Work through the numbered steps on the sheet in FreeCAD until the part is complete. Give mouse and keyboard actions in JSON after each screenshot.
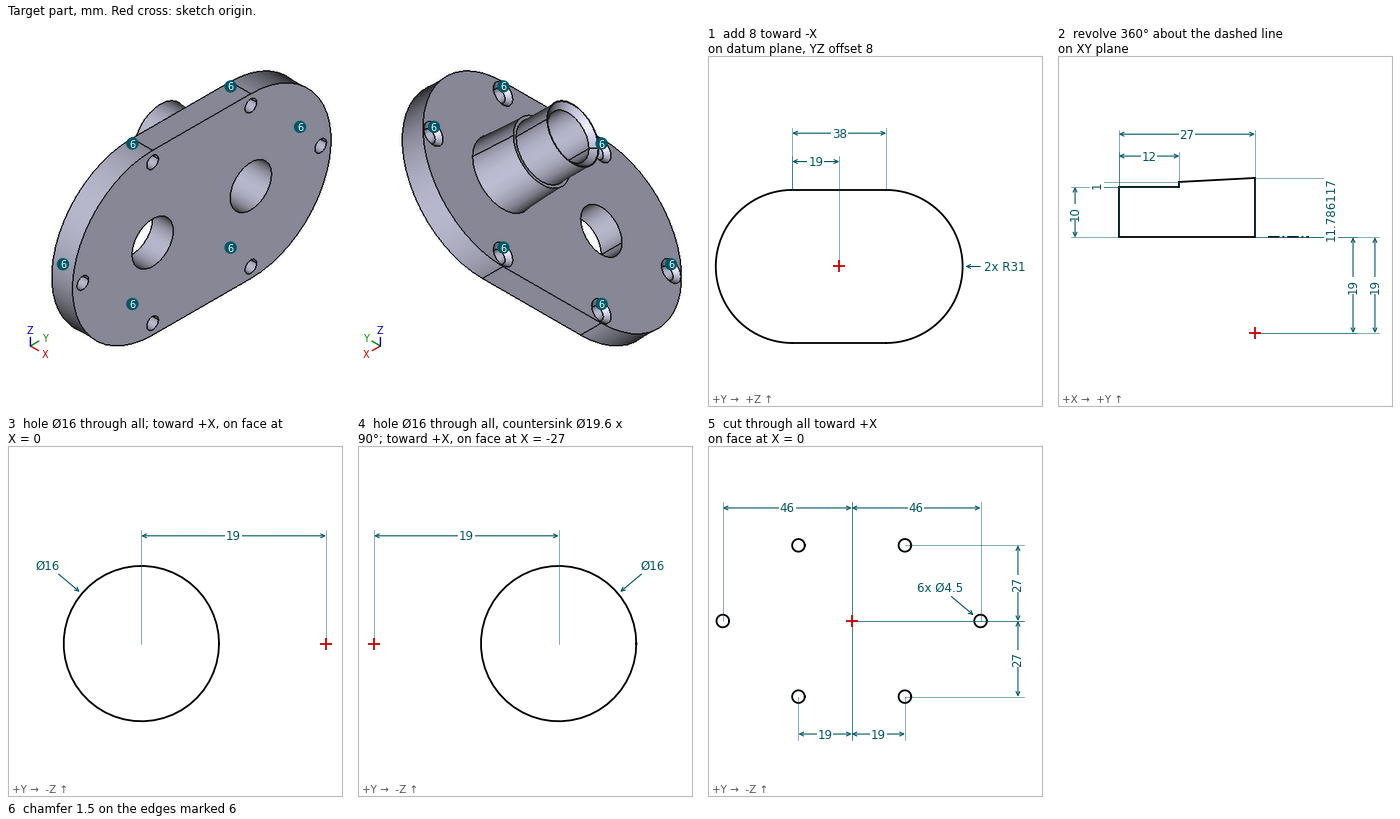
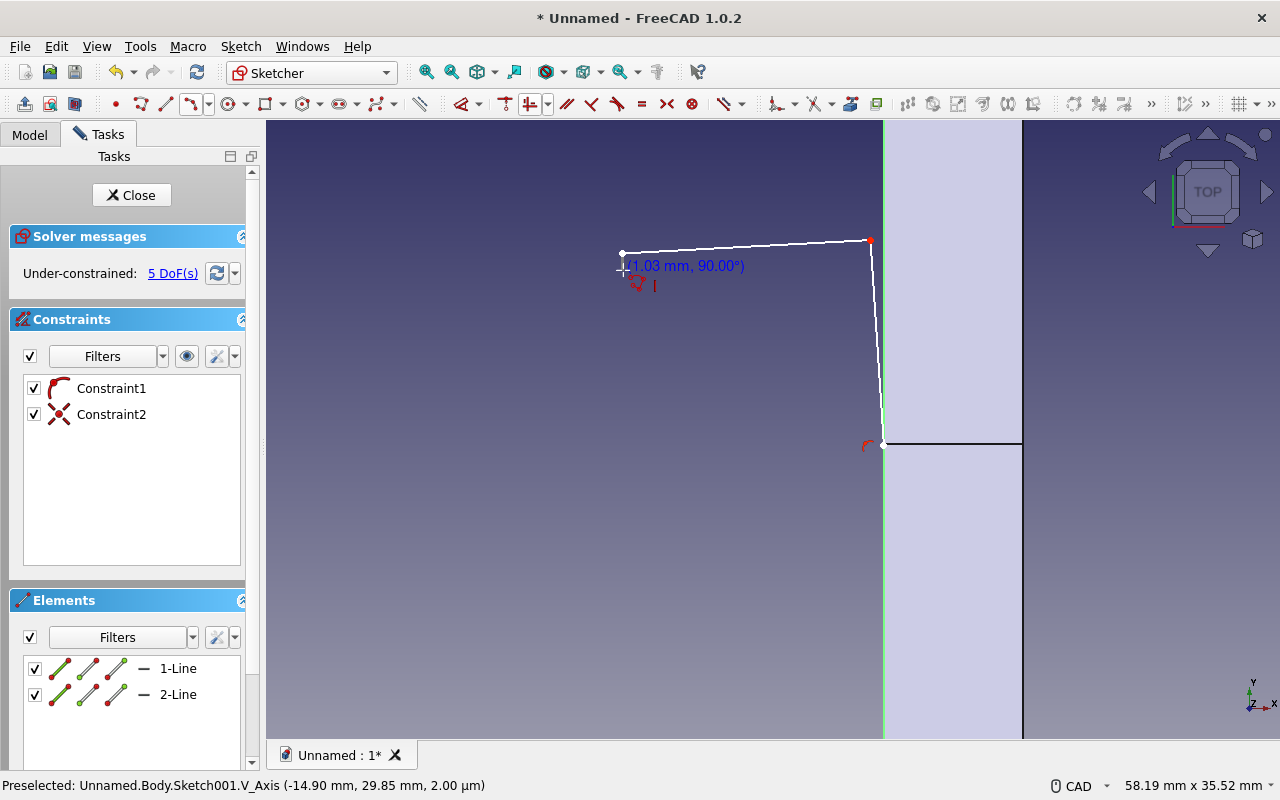
{"action": "left_click", "coordinate": [623, 270]}
{"action": "left_click", "coordinate": [413, 270]}
{"action": "left_click", "coordinate": [413, 444]}
{"action": "left_click", "coordinate": [884, 446]}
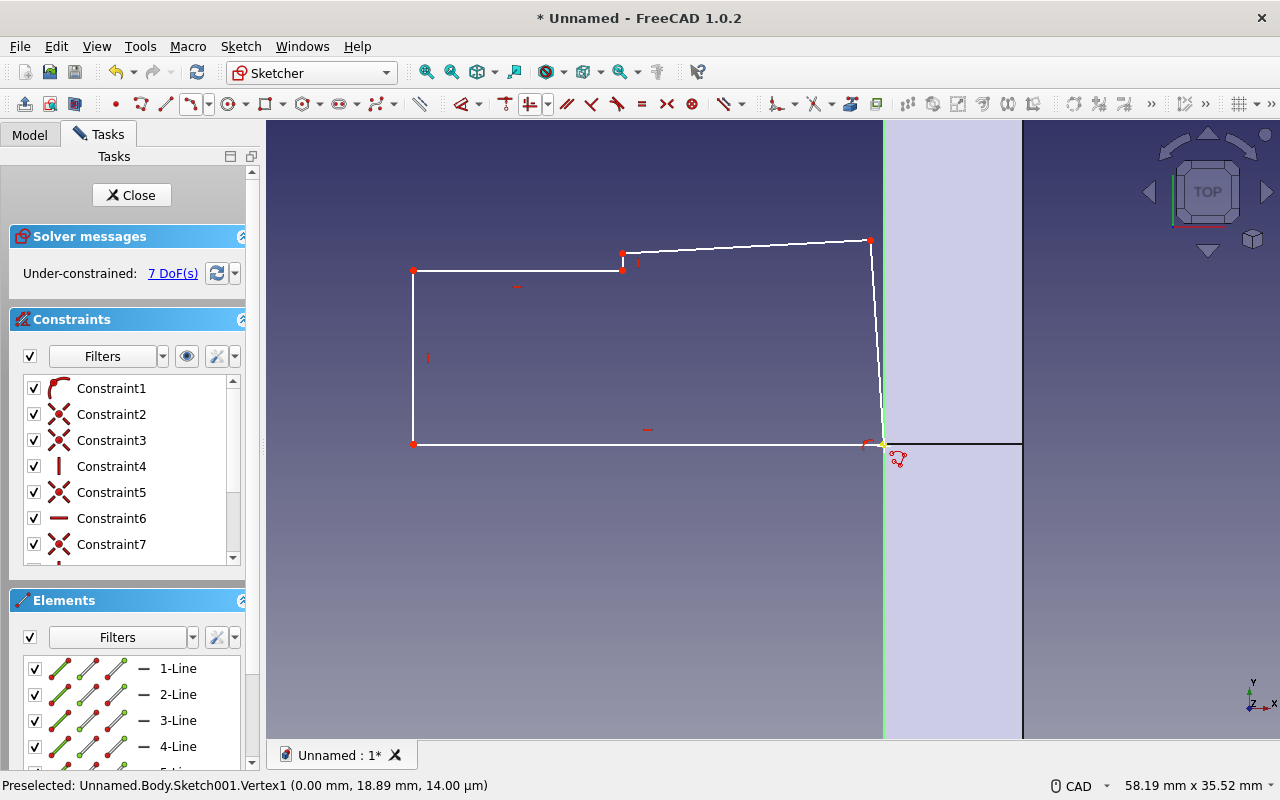
{"action": "key", "text": "g l"}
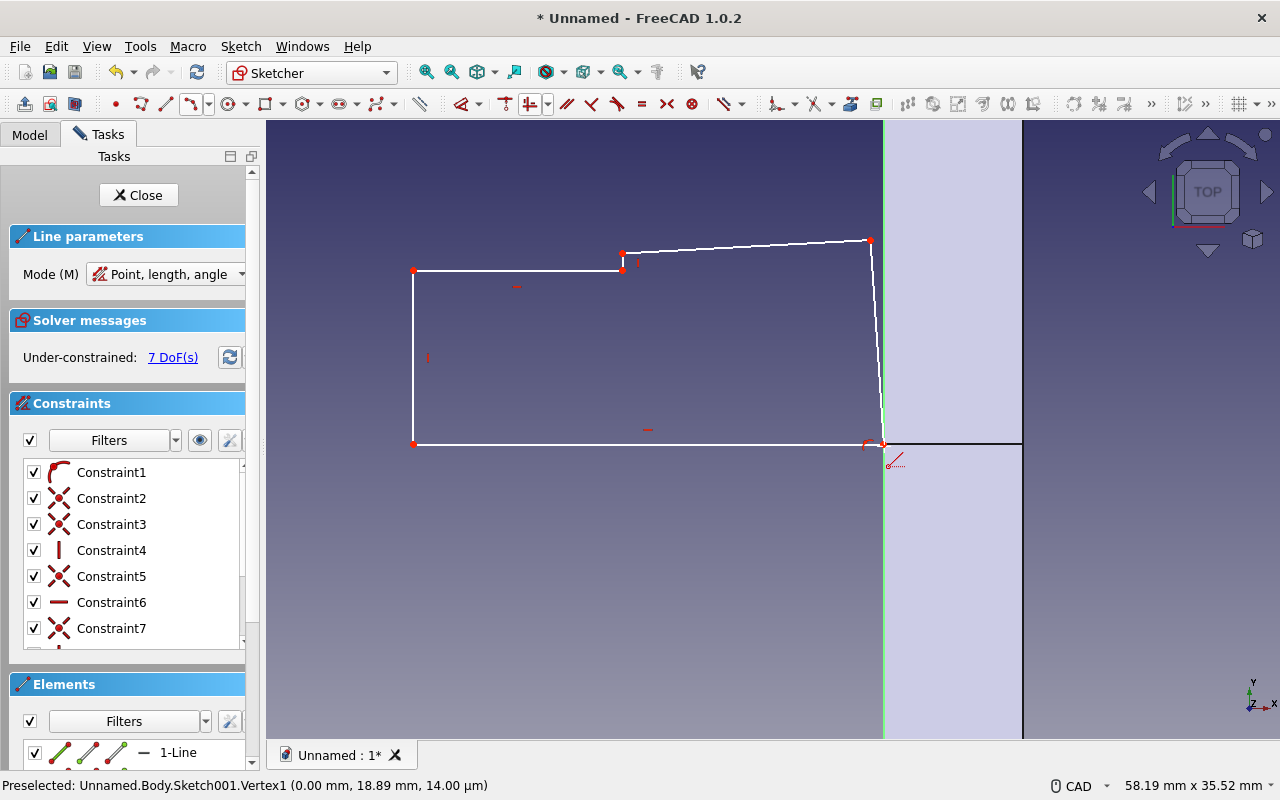
{"action": "left_click", "coordinate": [931, 444]}
{"action": "left_click", "coordinate": [1072, 444]}
{"action": "key", "text": "Escape"}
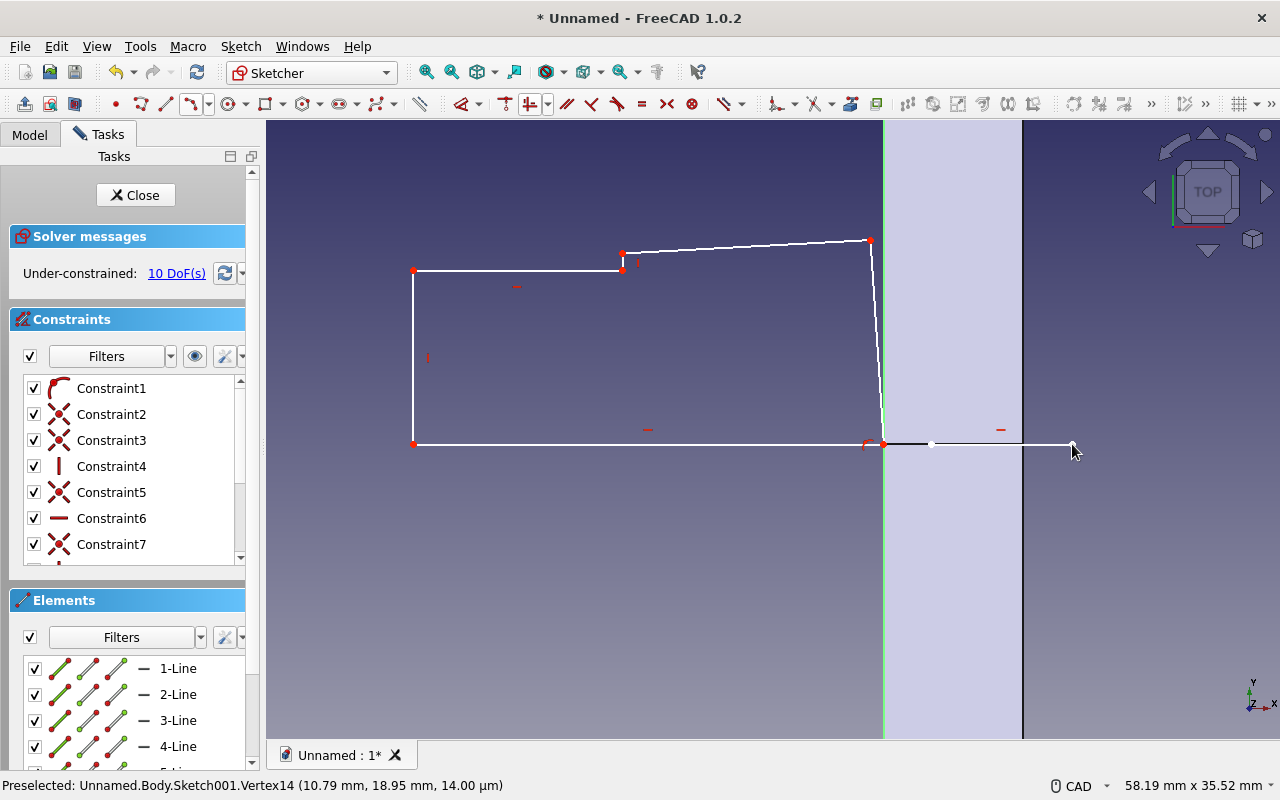
{"action": "left_click", "coordinate": [973, 445]}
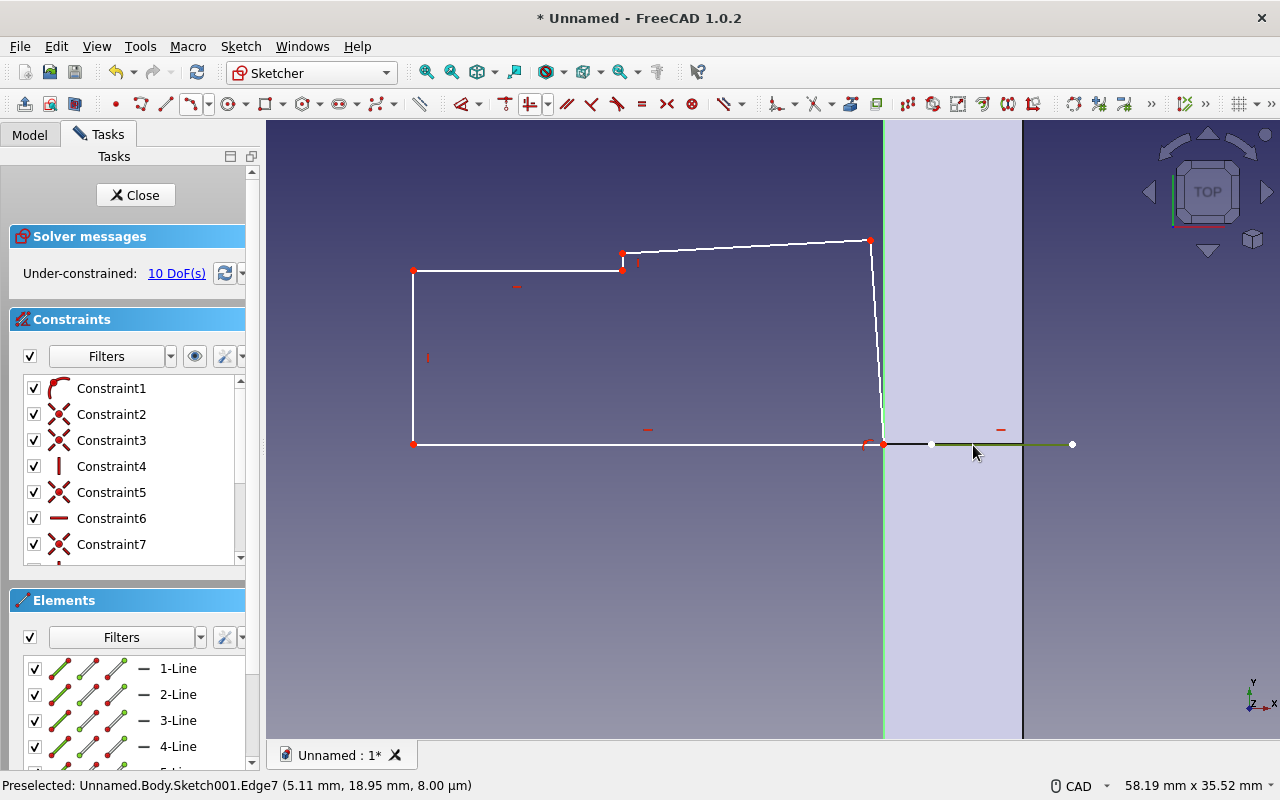
{"action": "left_click", "coordinate": [420, 104]}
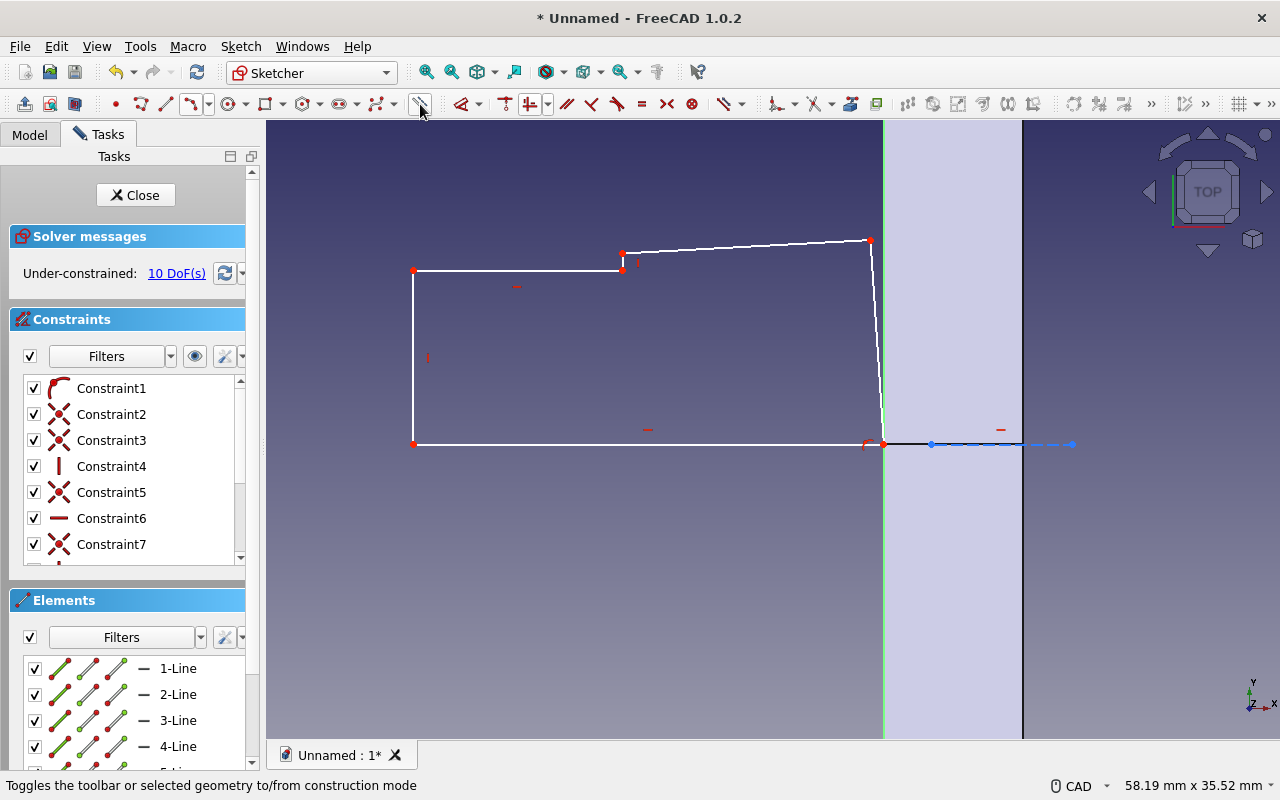
{"action": "scroll", "coordinate": [875, 302], "scroll_direction": "up", "scroll_amount": 2}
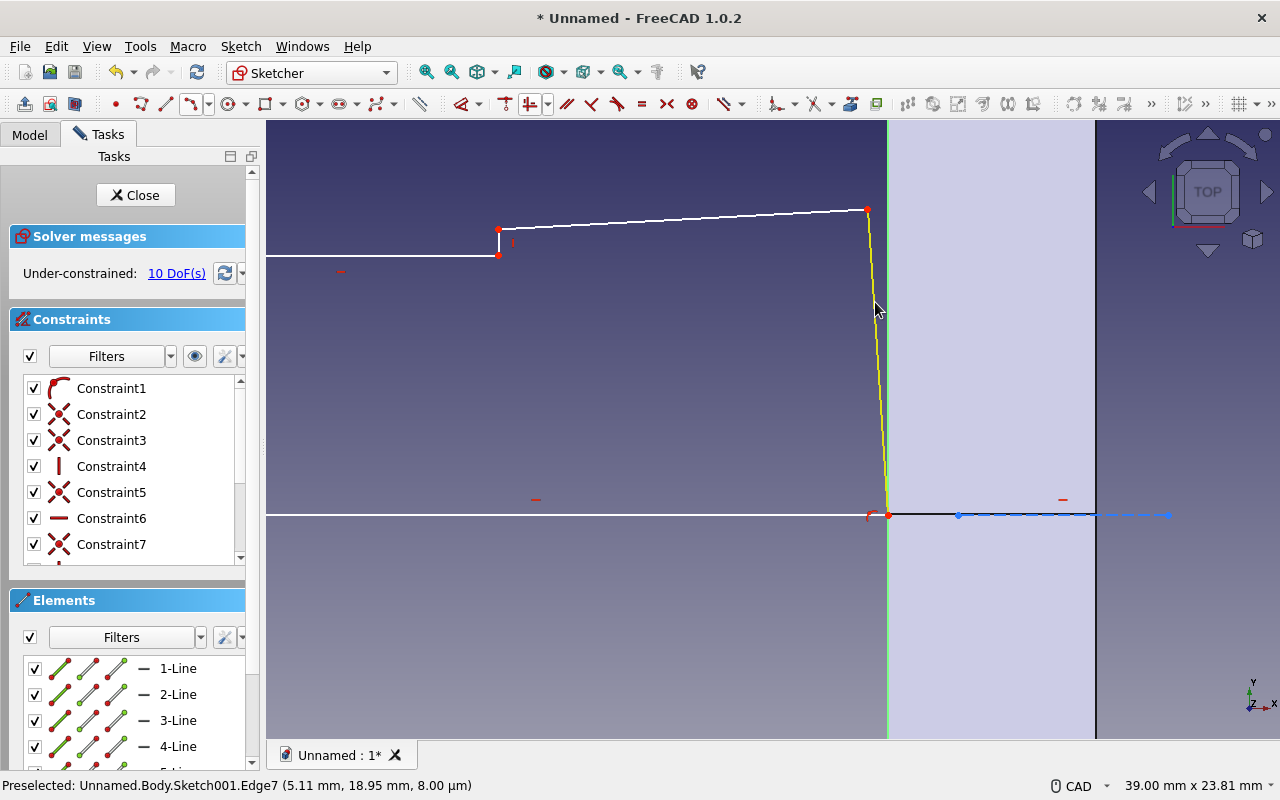
{"action": "left_click", "coordinate": [874, 301]}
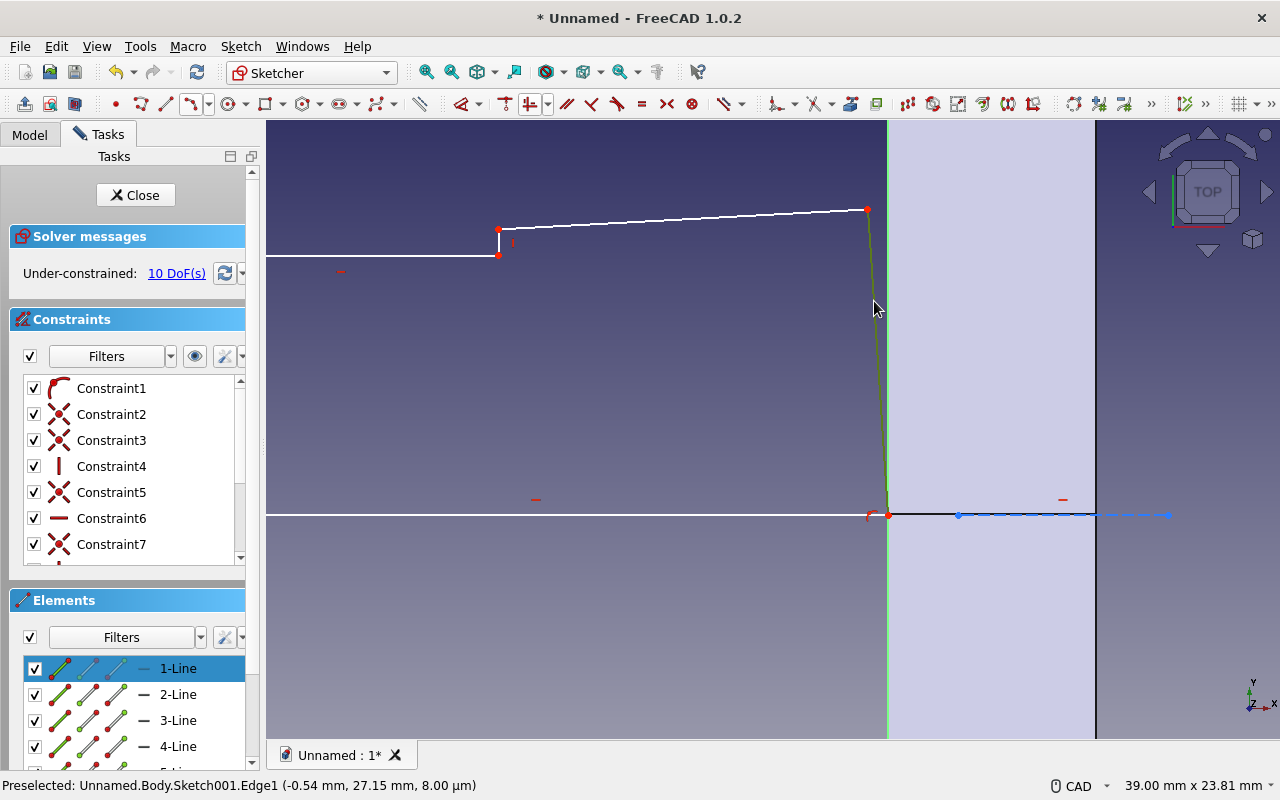
{"action": "left_click", "coordinate": [548, 104]}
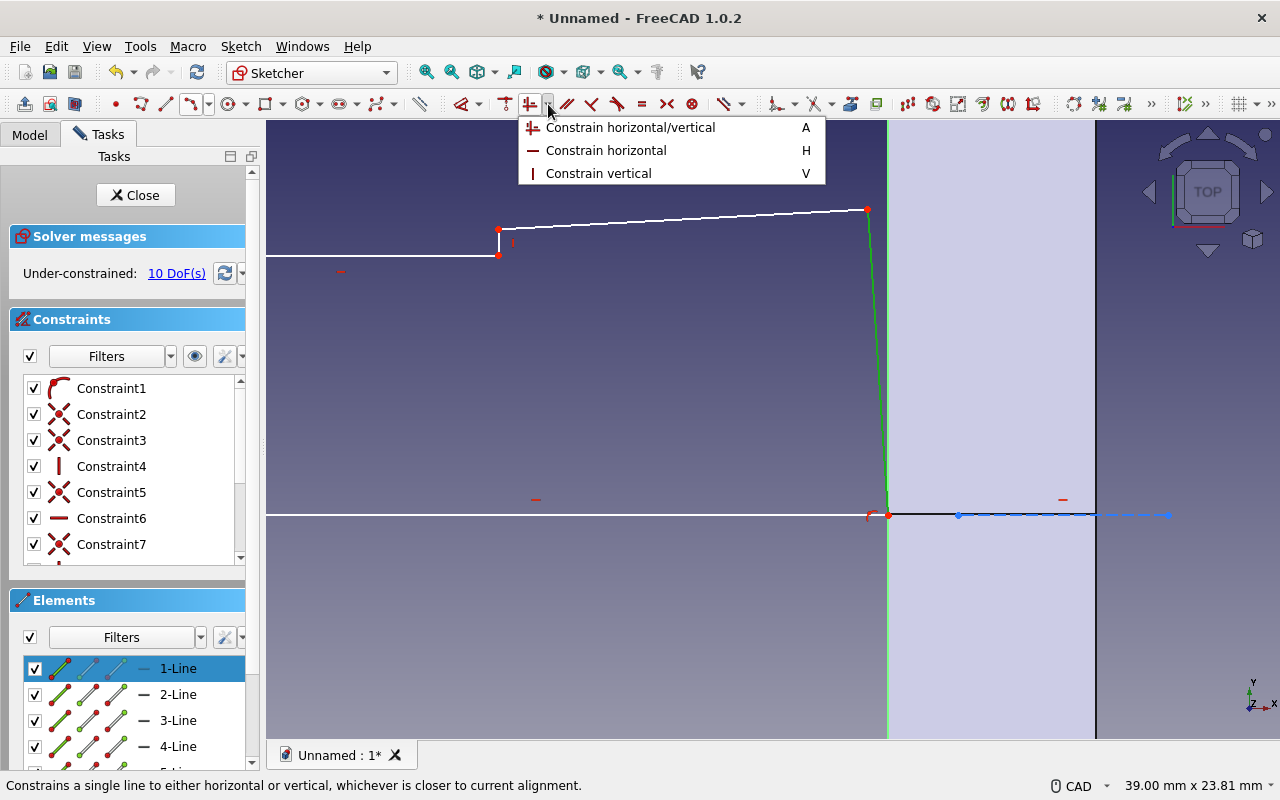
{"action": "left_click", "coordinate": [672, 174]}